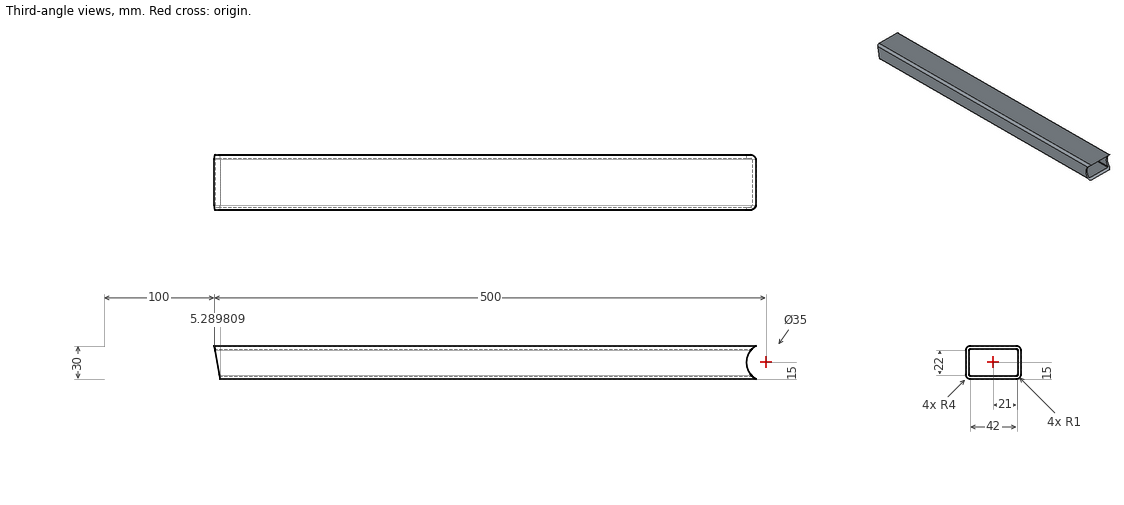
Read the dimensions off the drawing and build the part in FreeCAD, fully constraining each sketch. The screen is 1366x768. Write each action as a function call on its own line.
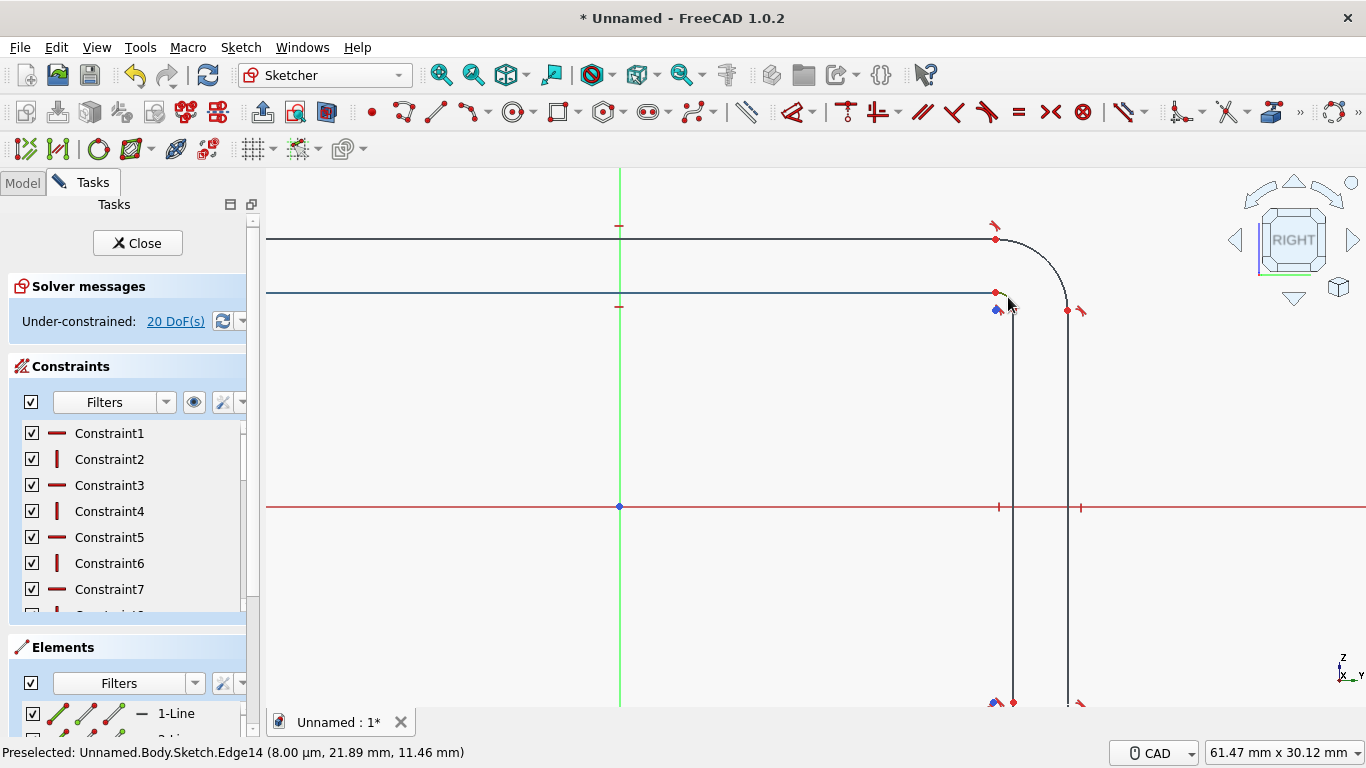
key(t)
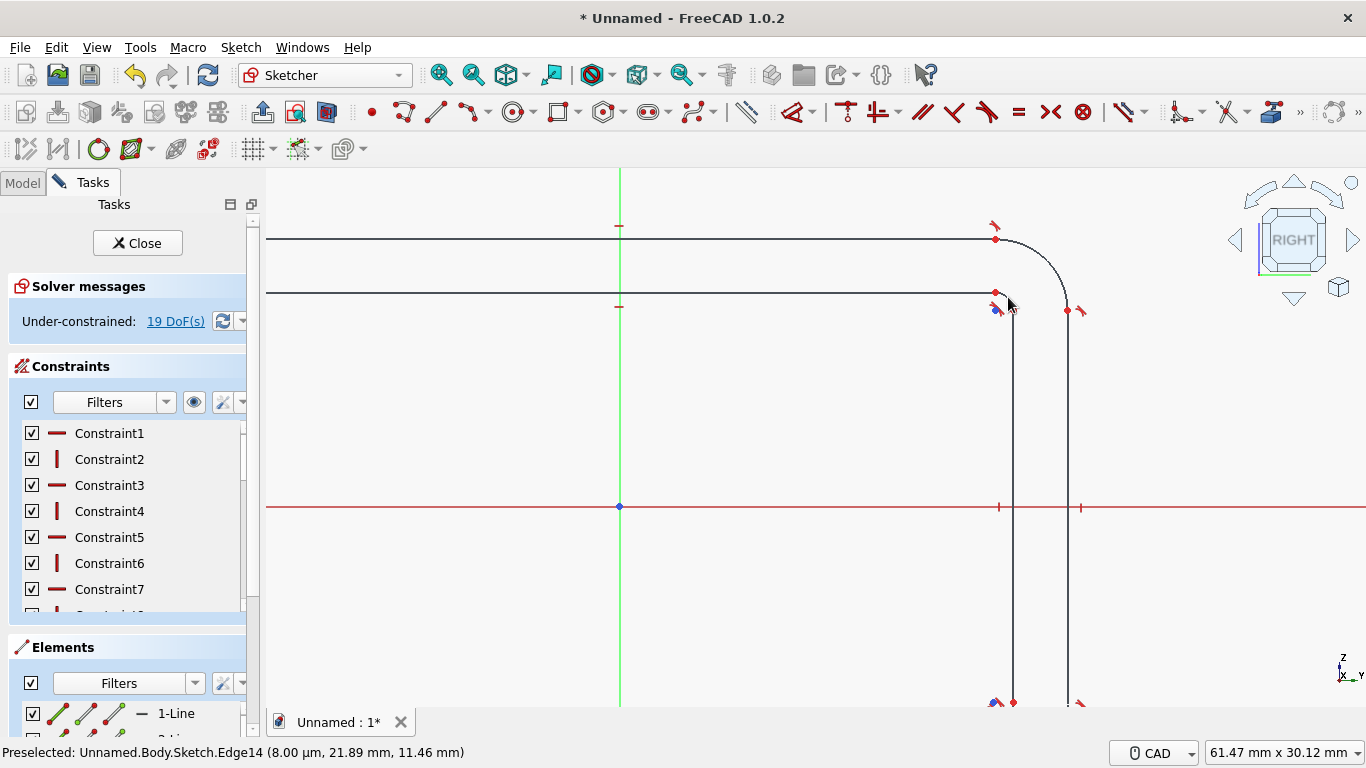
click(770, 293)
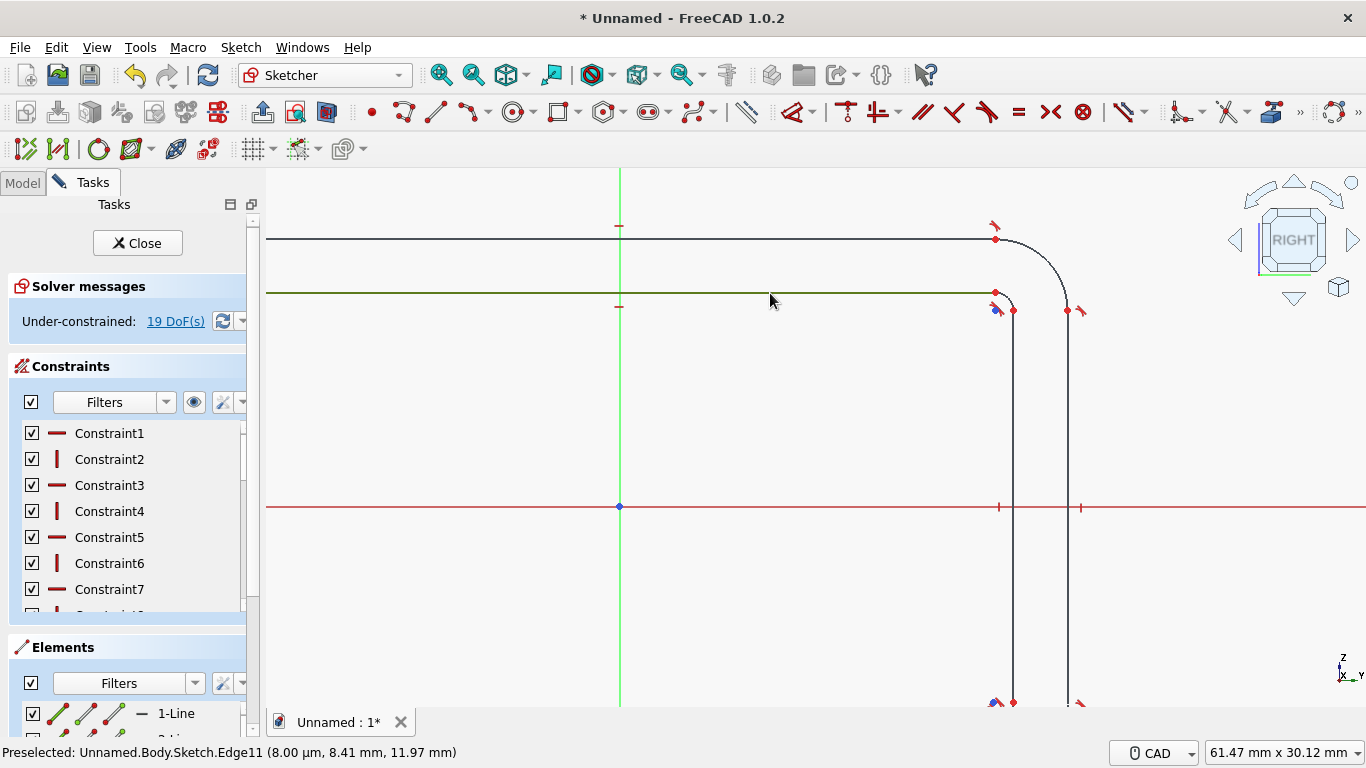
scroll(1008, 297, down, 2)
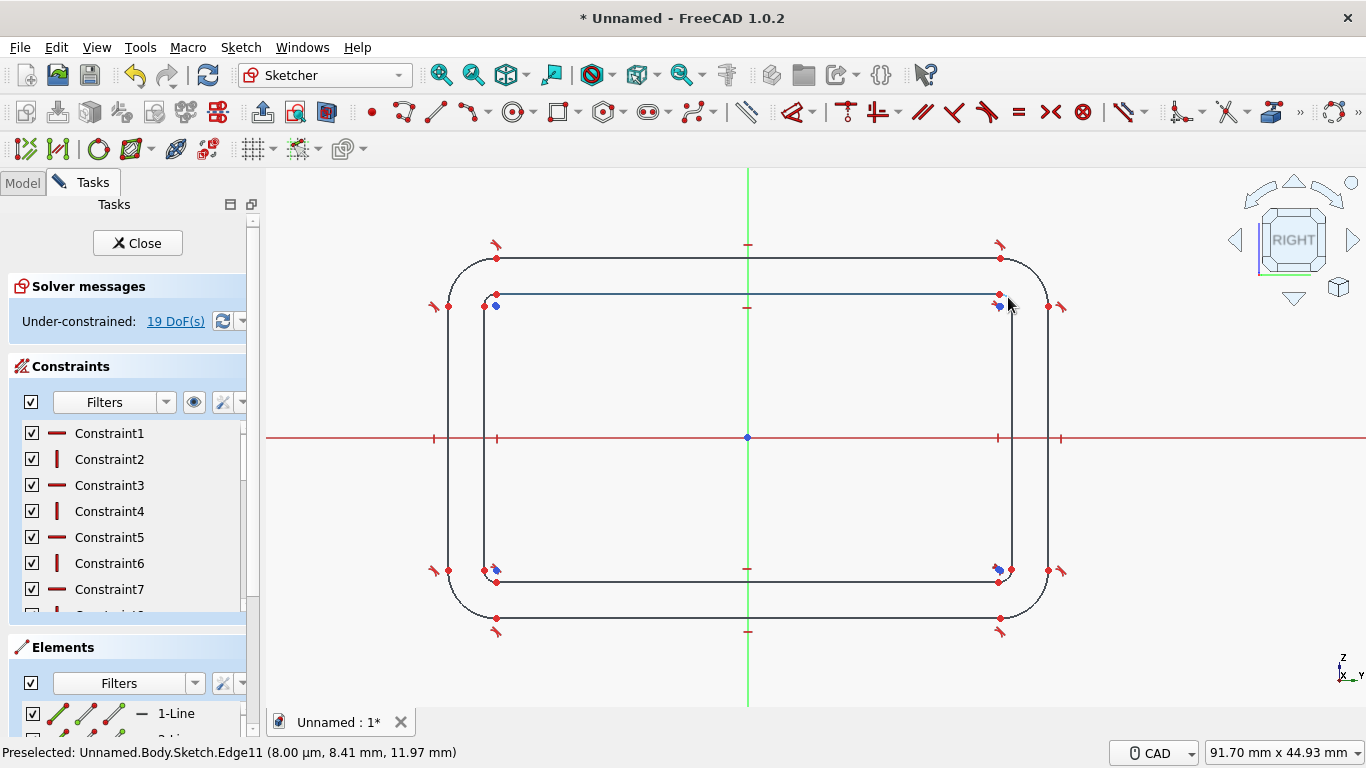
scroll(487, 298, up, 2)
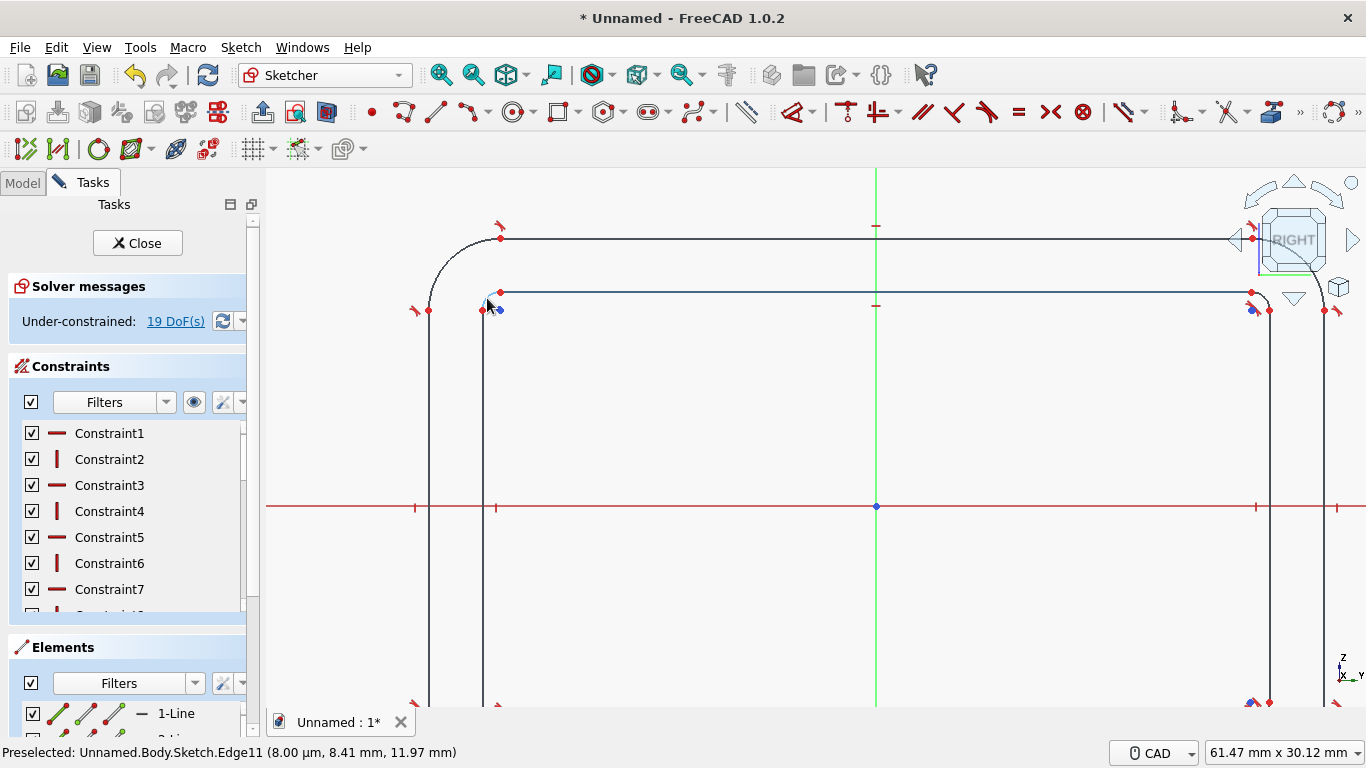
click(488, 297)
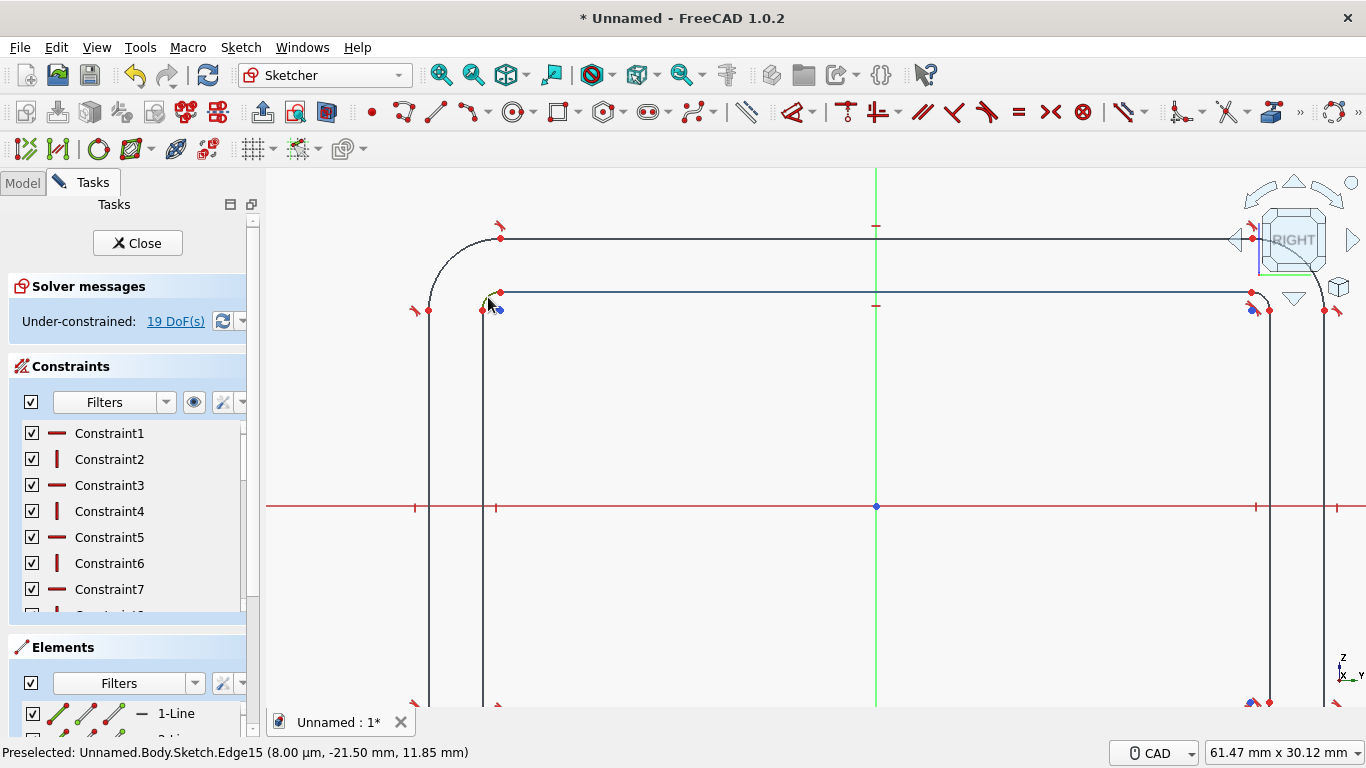
key(t)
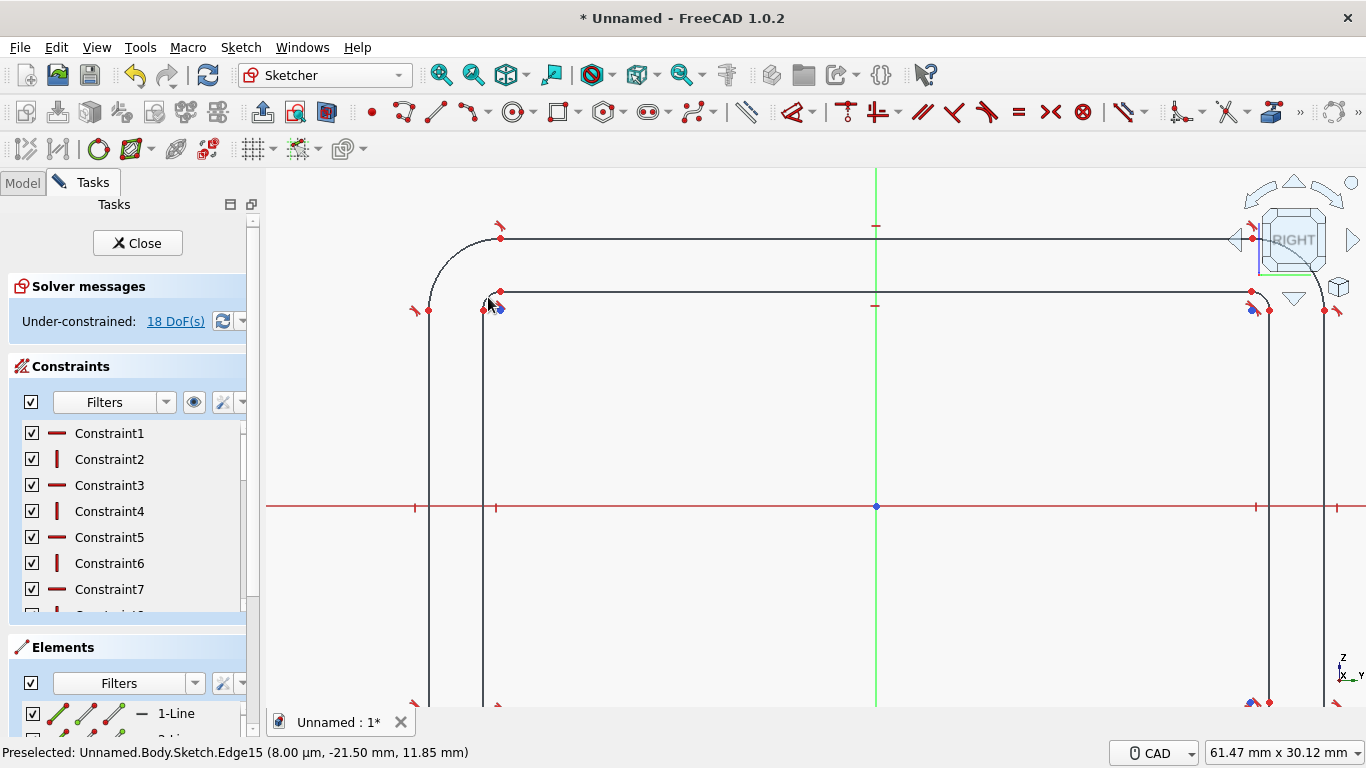
click(483, 429)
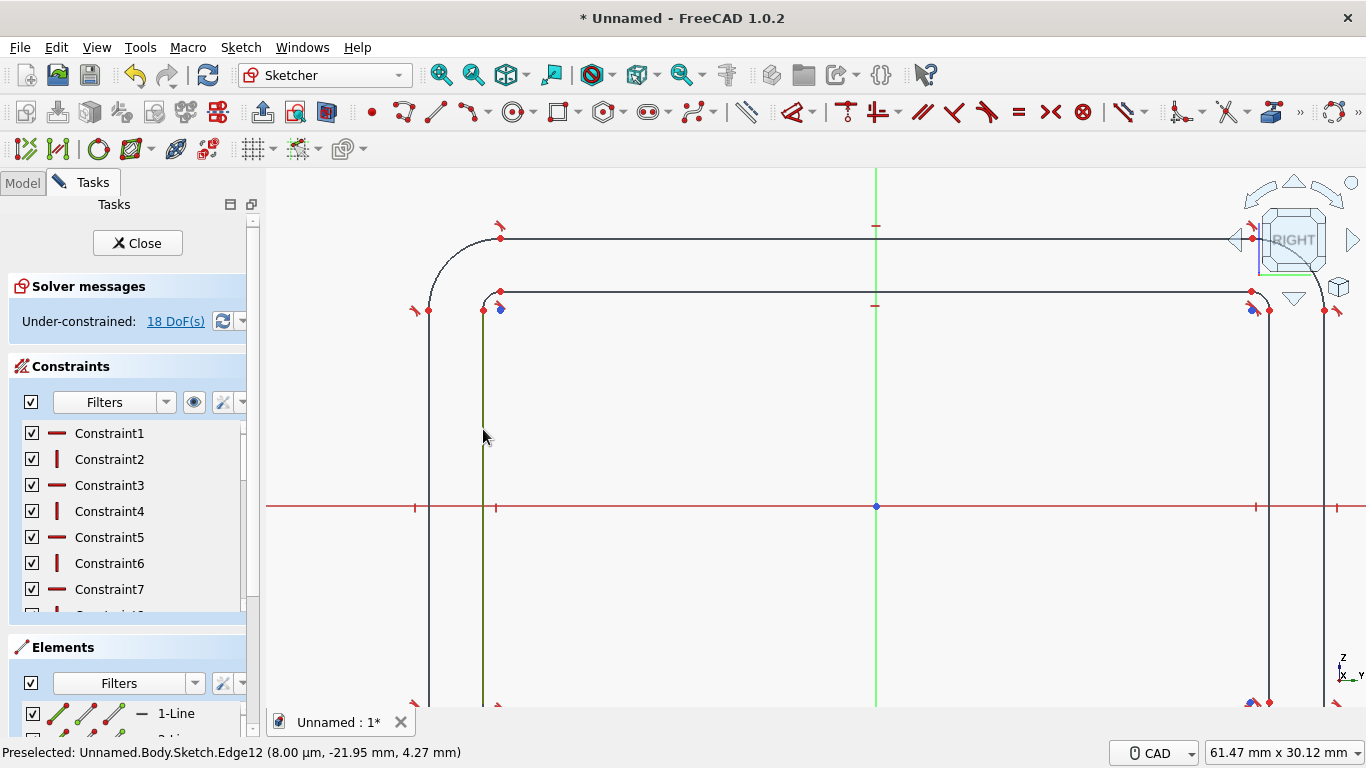
click(488, 297)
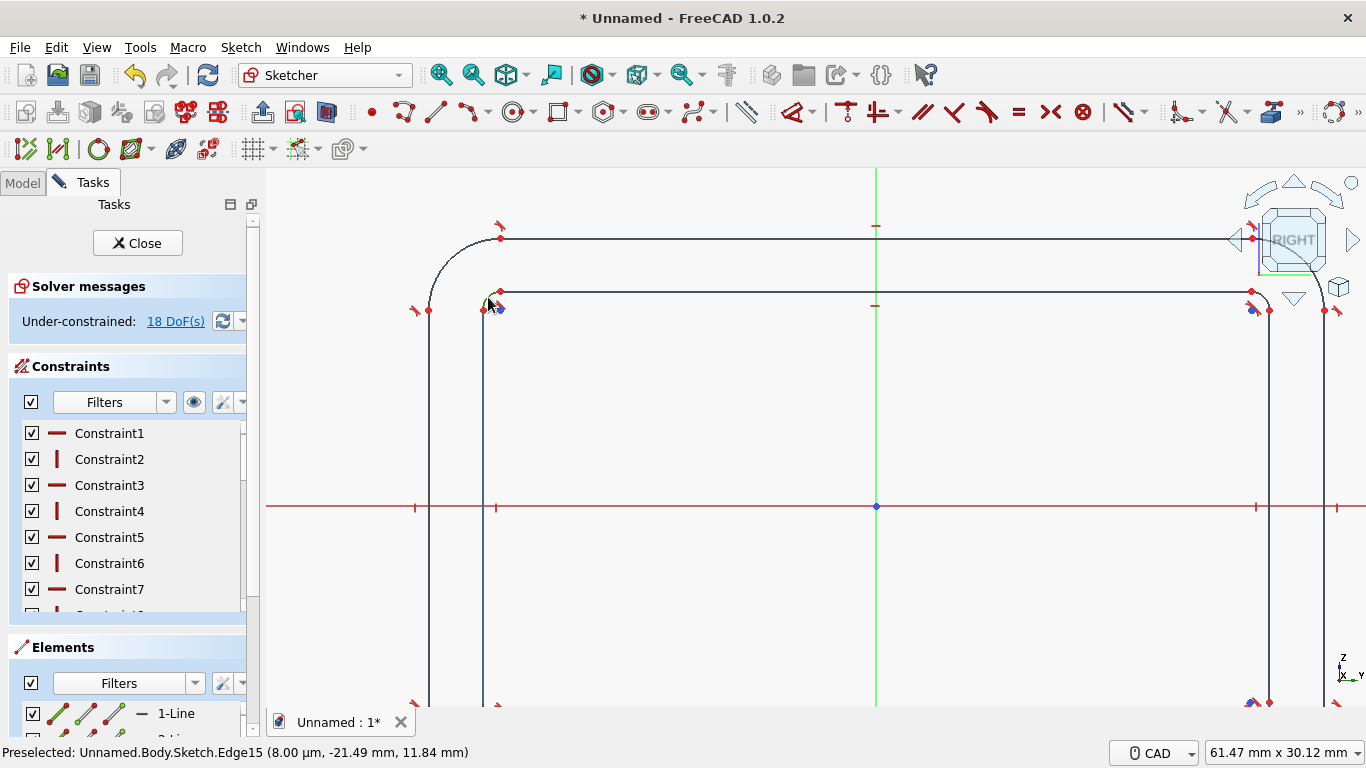
key(t)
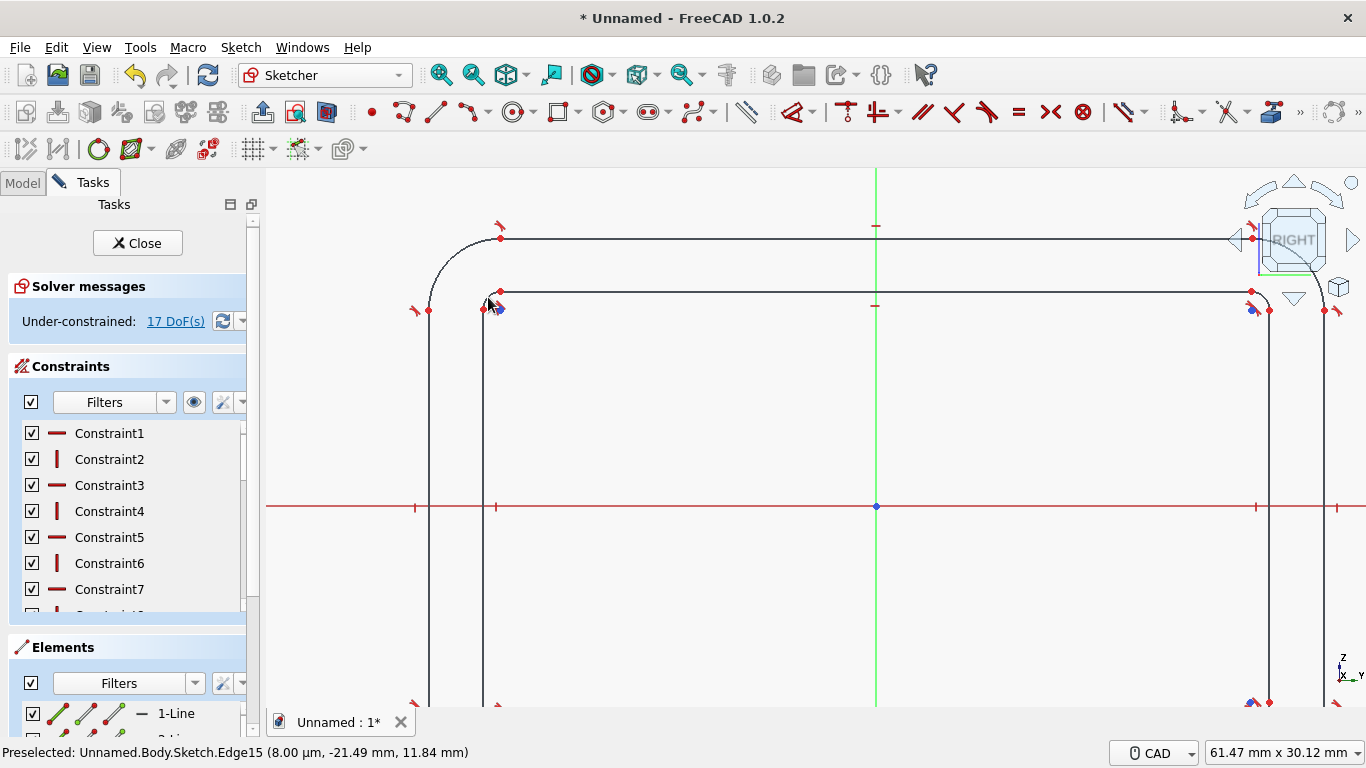
click(483, 428)